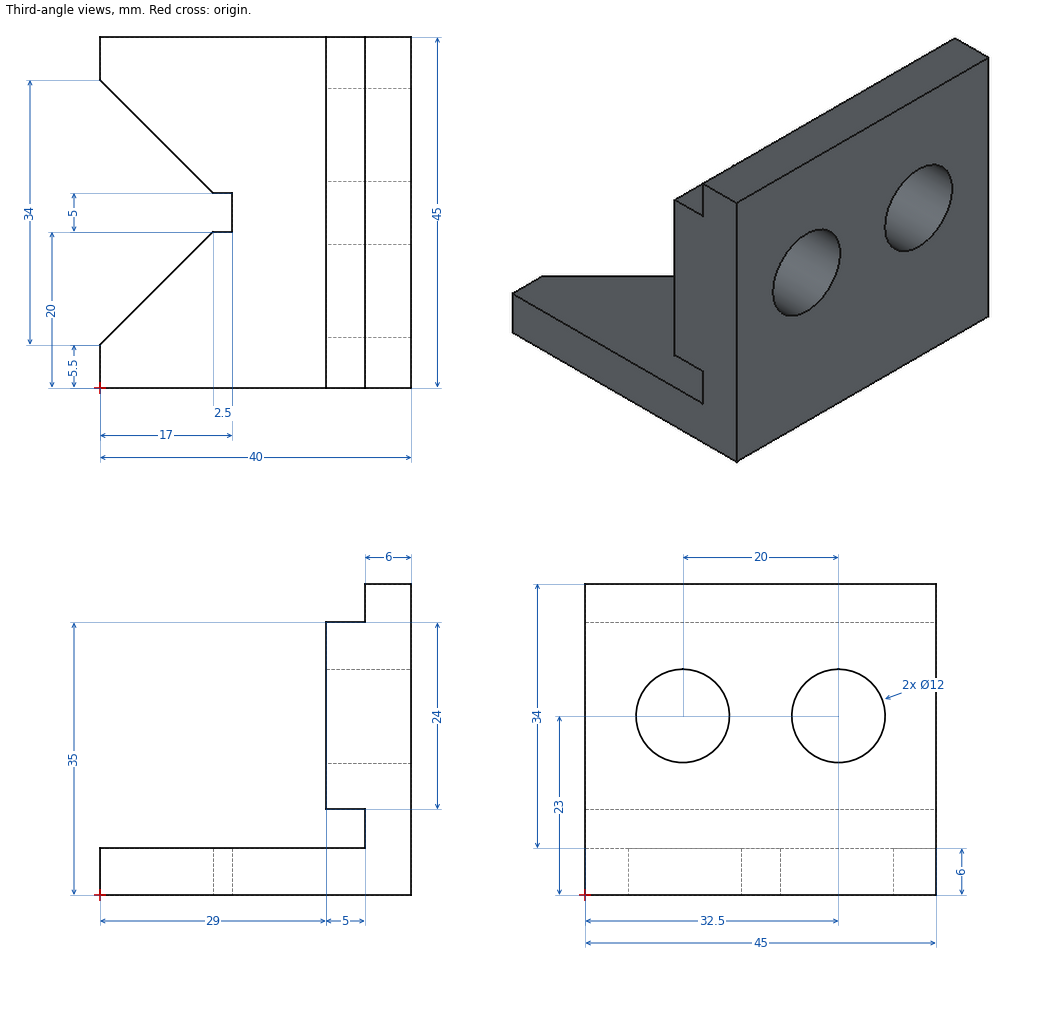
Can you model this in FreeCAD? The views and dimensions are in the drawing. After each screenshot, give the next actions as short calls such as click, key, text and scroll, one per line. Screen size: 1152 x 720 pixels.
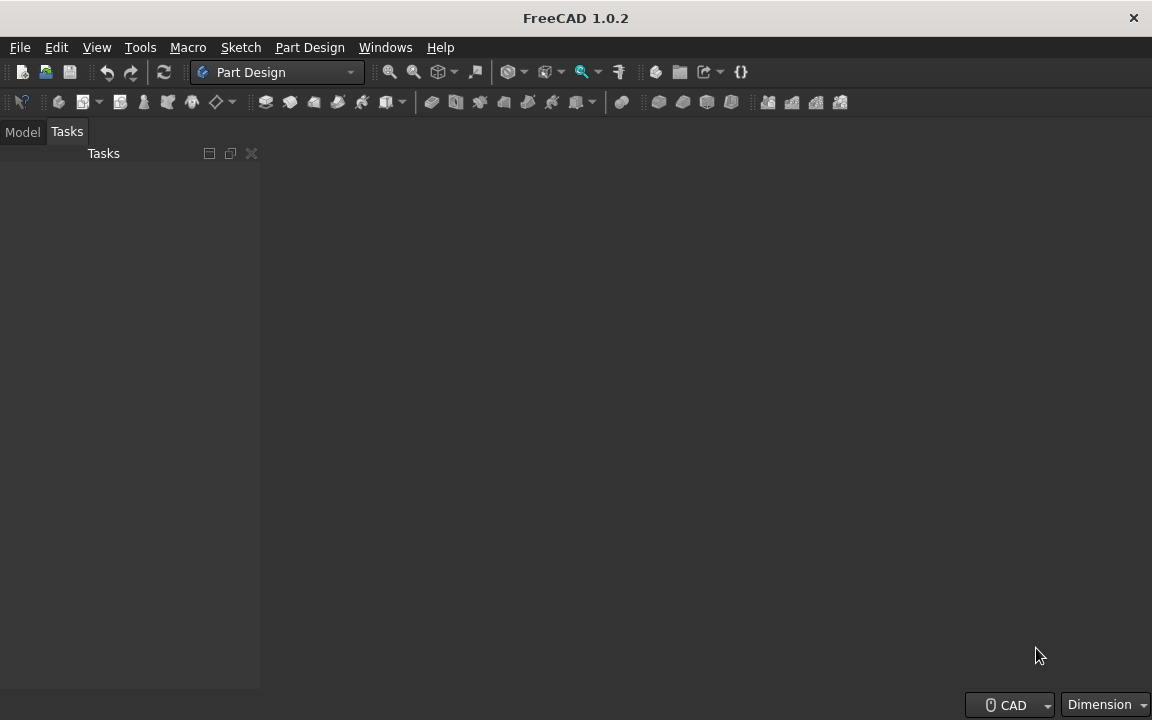
click(22, 72)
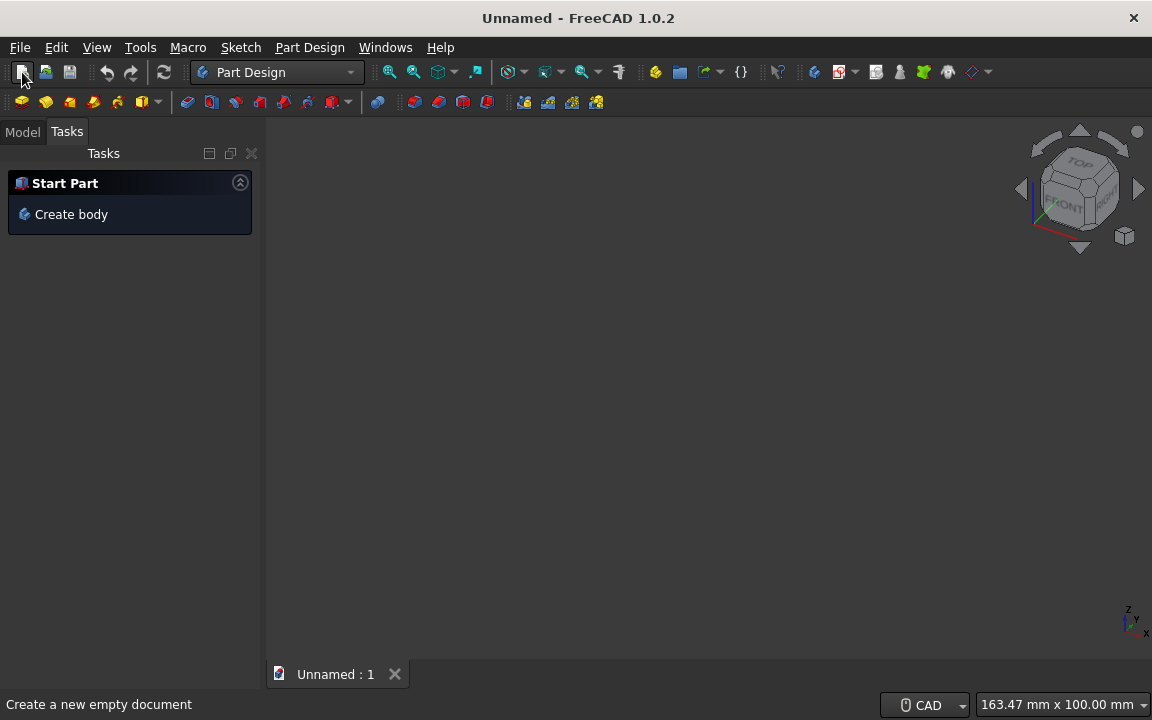
click(840, 72)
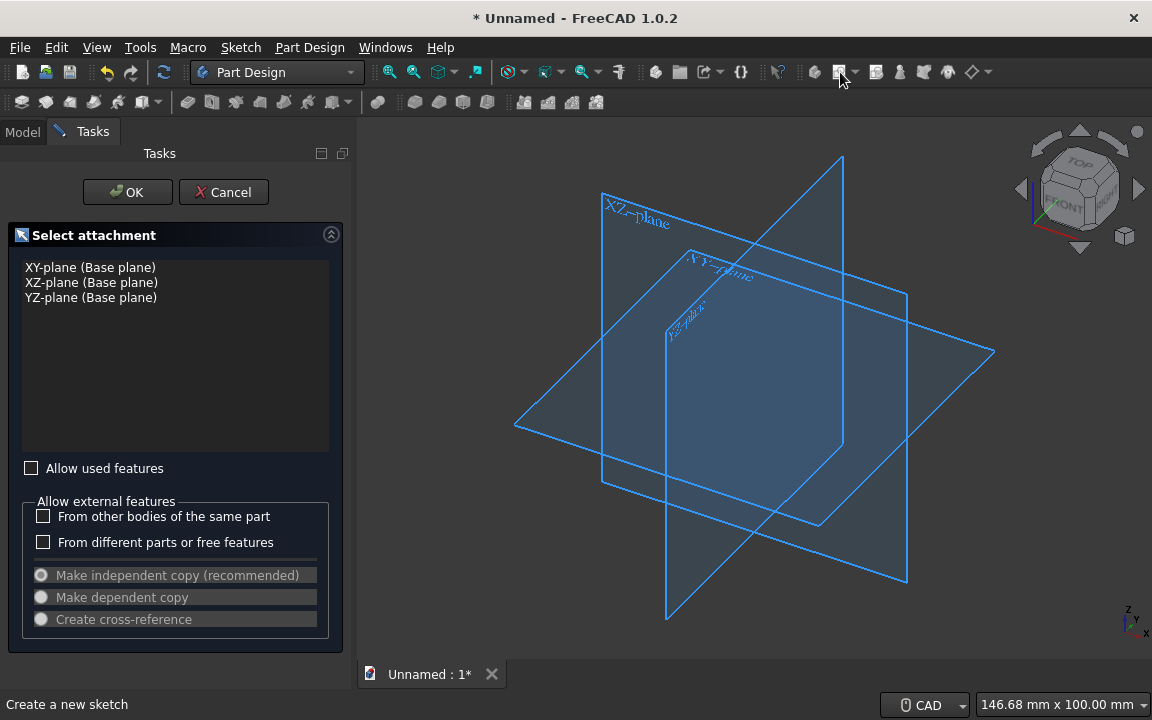
click(82, 268)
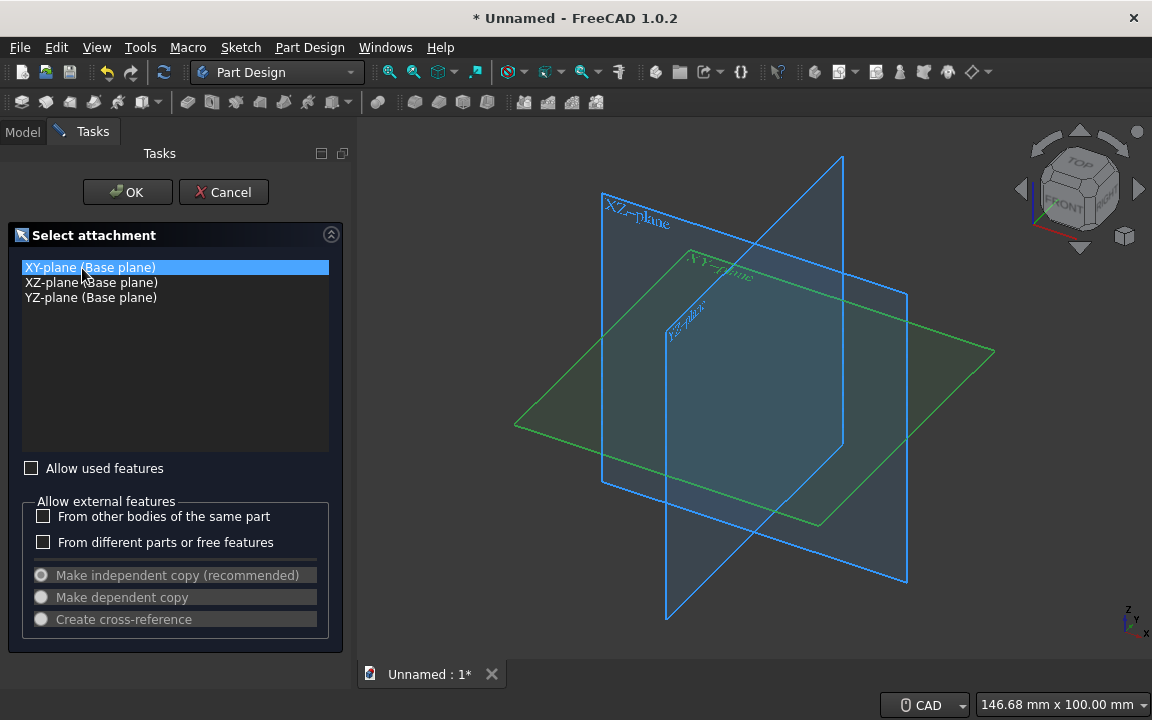
click(128, 192)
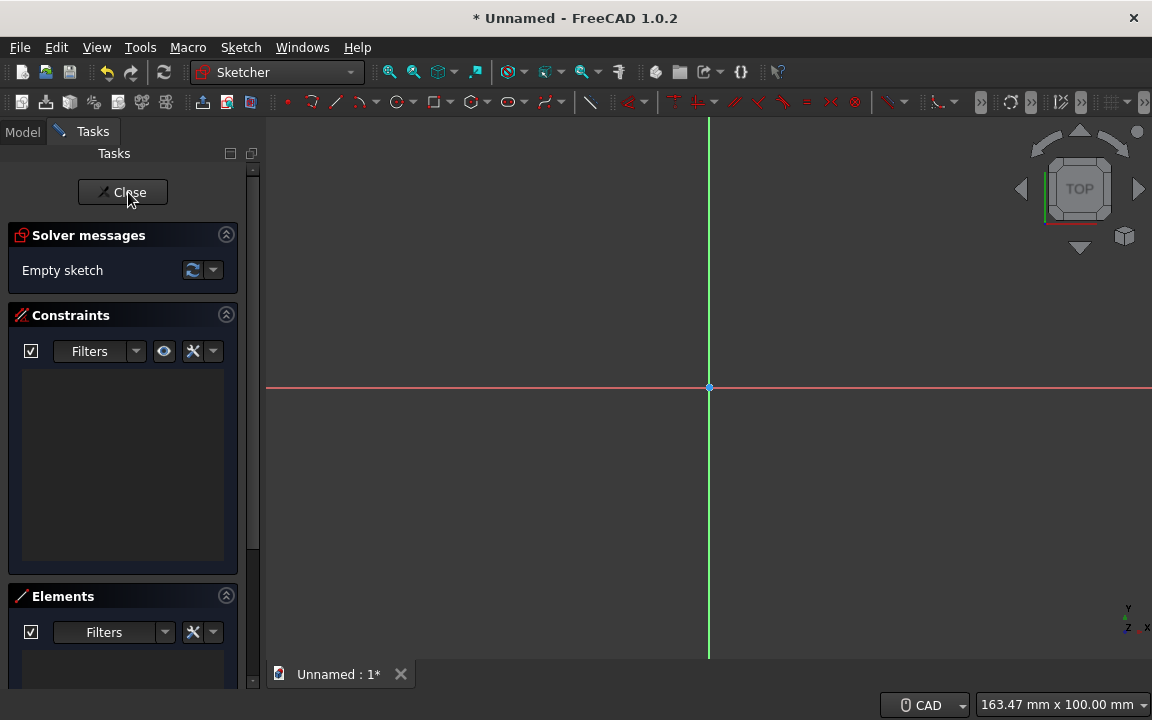
scroll(294, 631, down, 1)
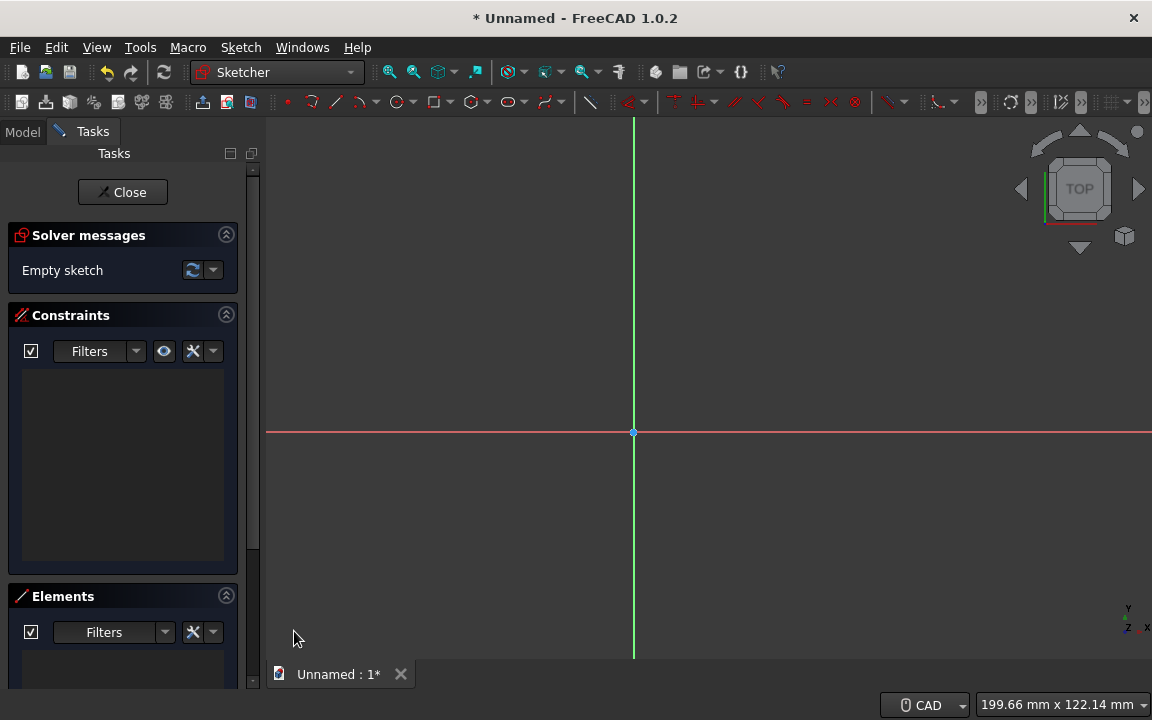
scroll(822, 265, up, 3)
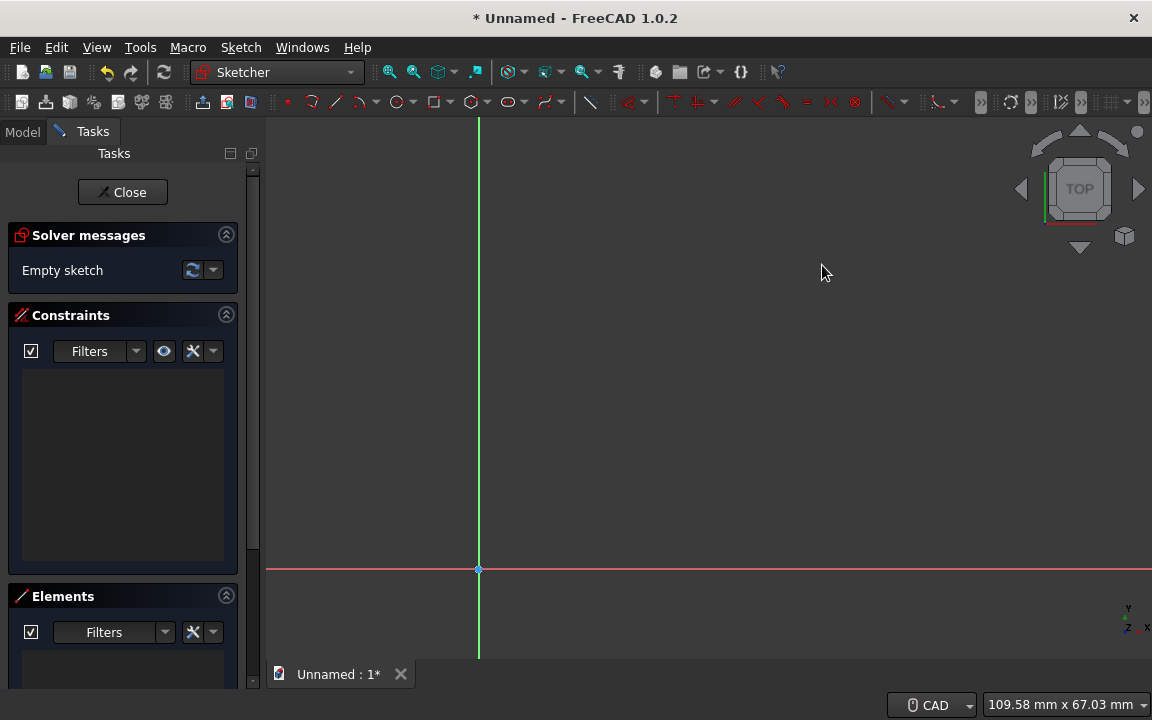
click(434, 102)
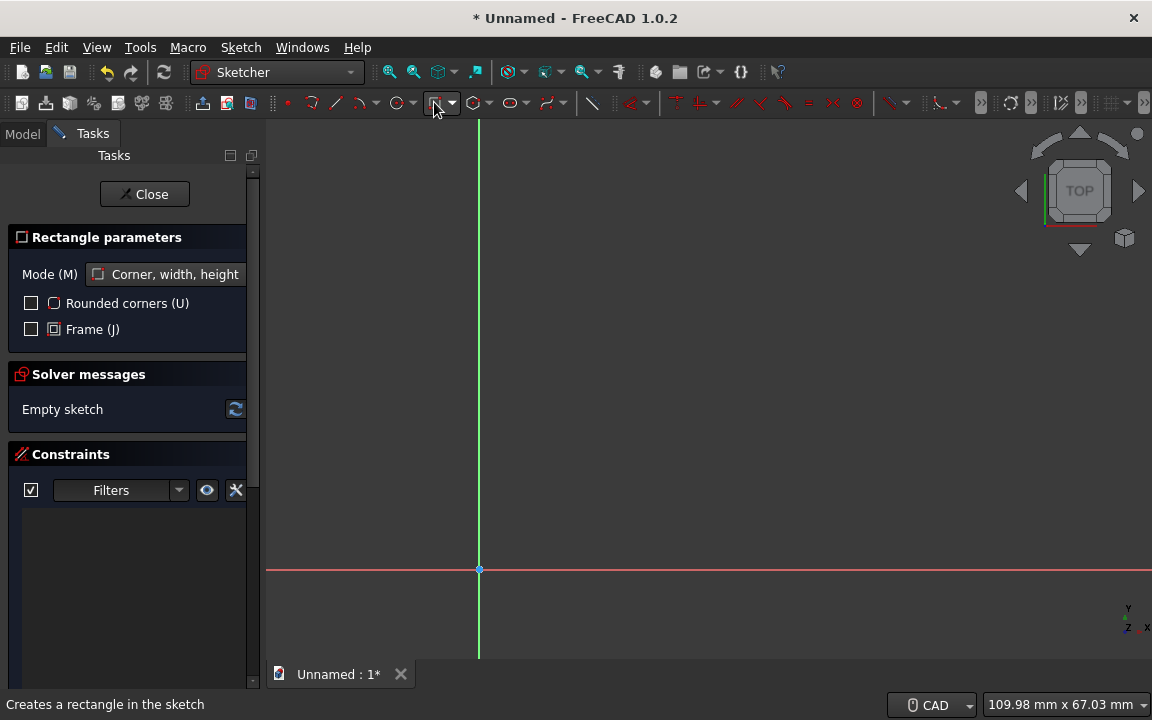
click(479, 570)
click(802, 207)
key(Escape)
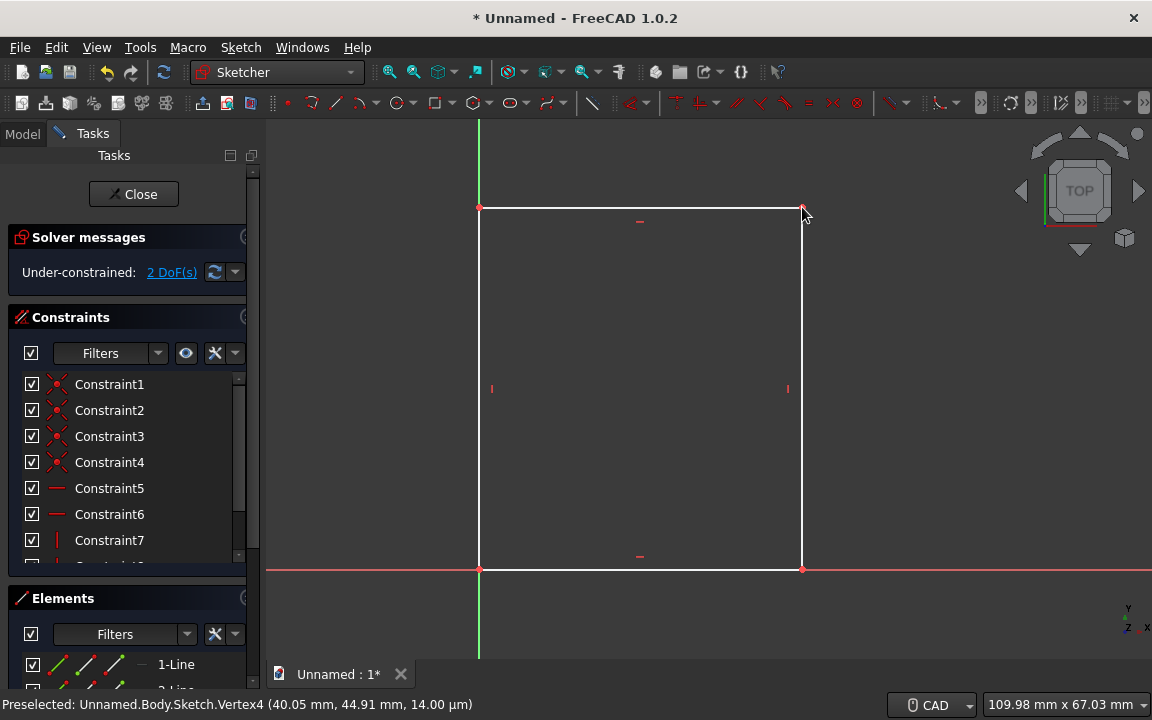
click(630, 104)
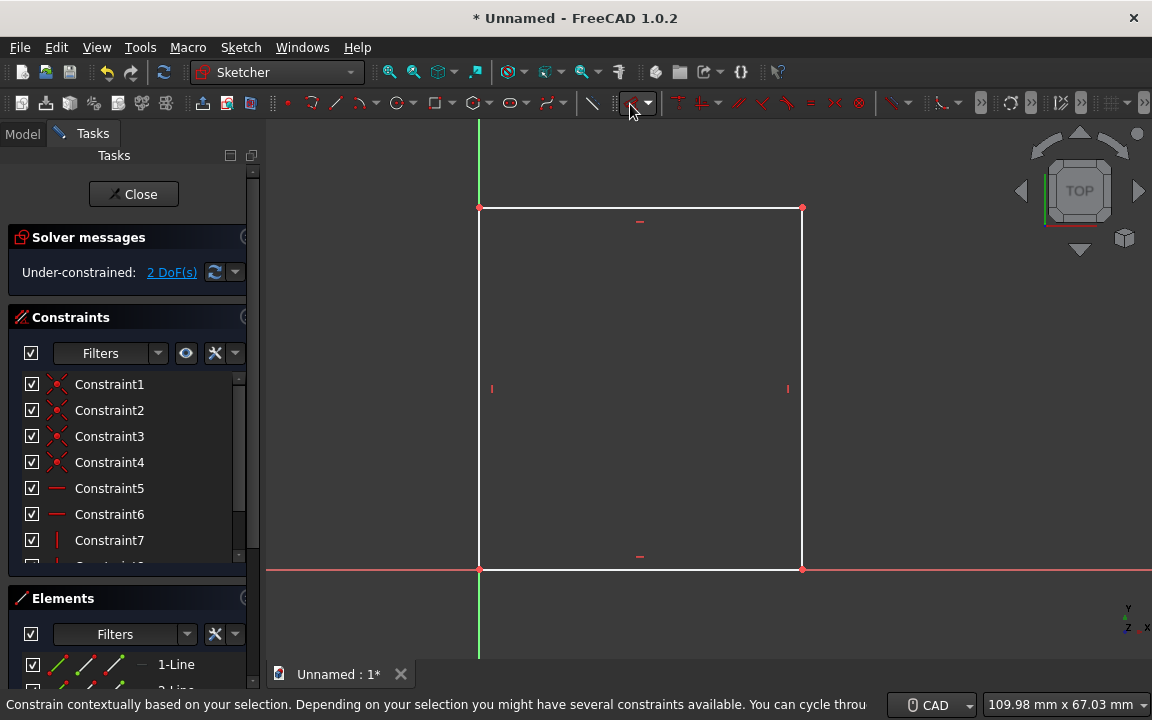
click(576, 570)
click(641, 604)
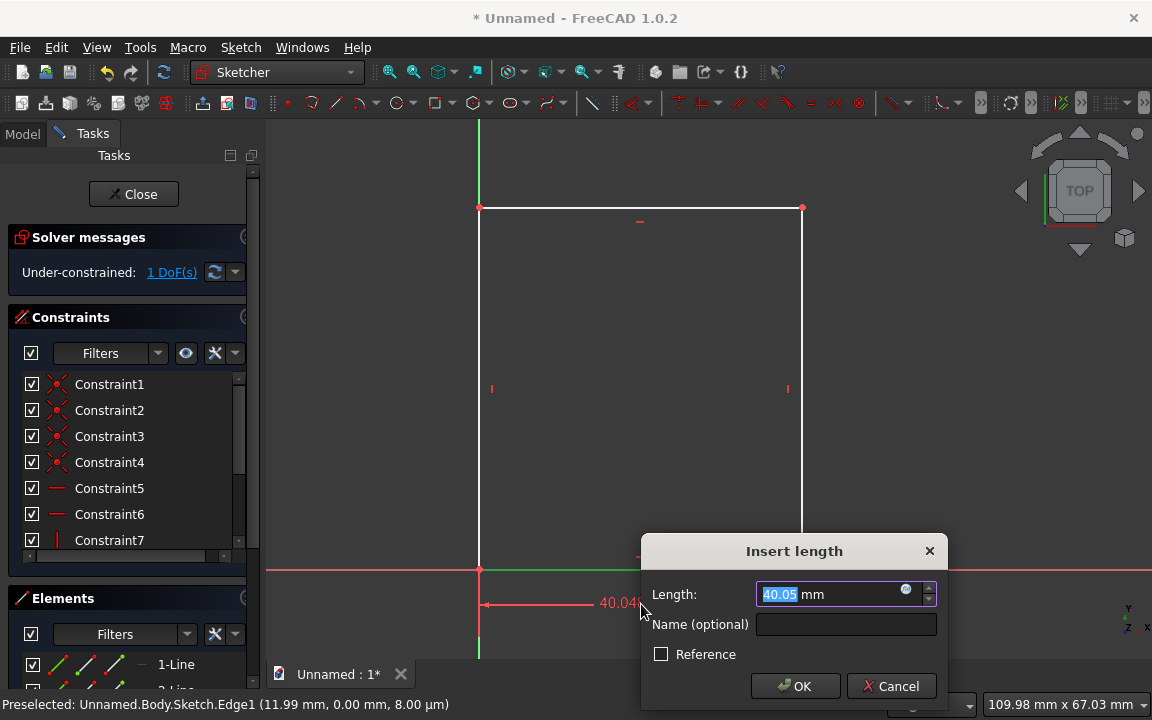
text(40)
key(Return)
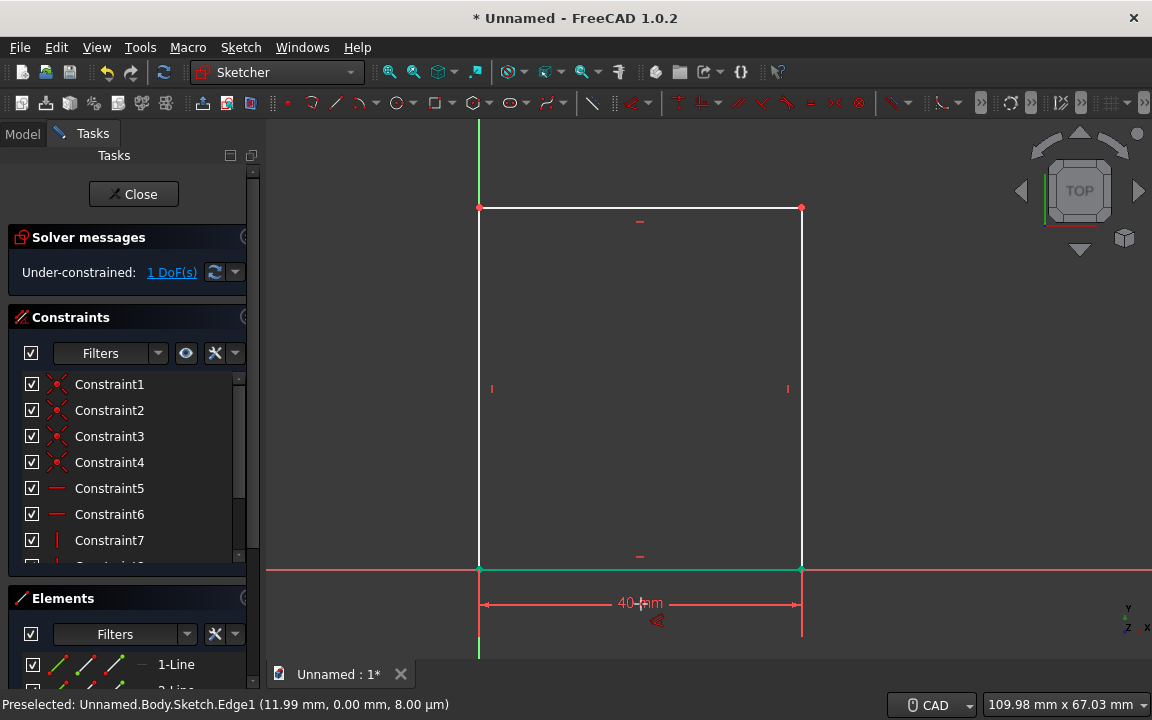
click(802, 461)
click(836, 389)